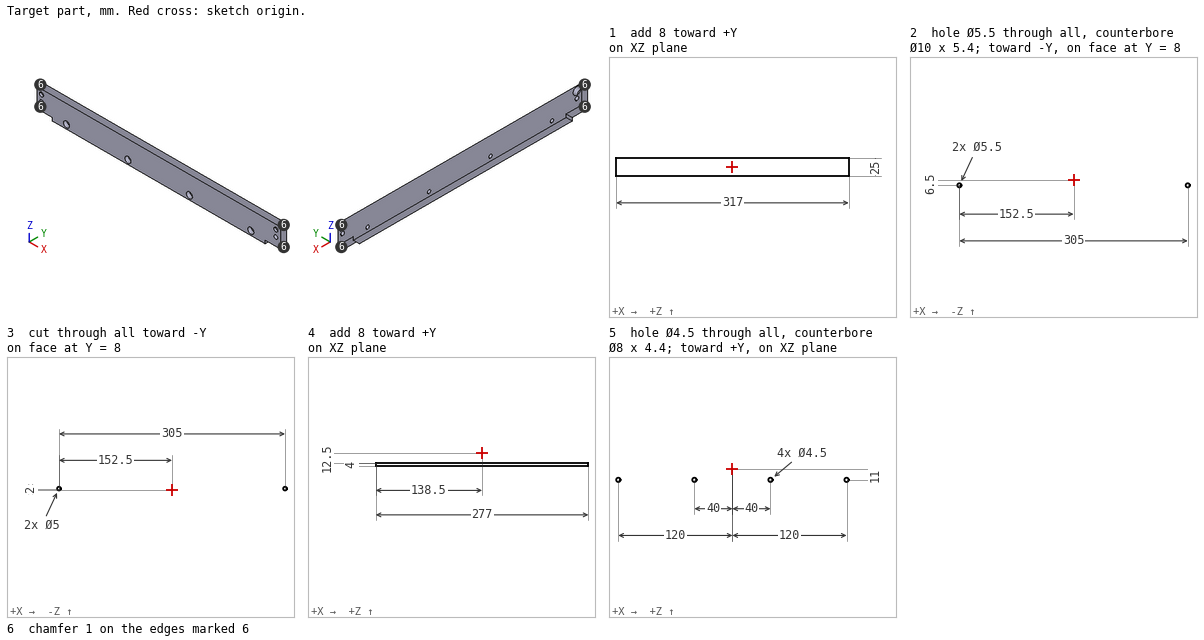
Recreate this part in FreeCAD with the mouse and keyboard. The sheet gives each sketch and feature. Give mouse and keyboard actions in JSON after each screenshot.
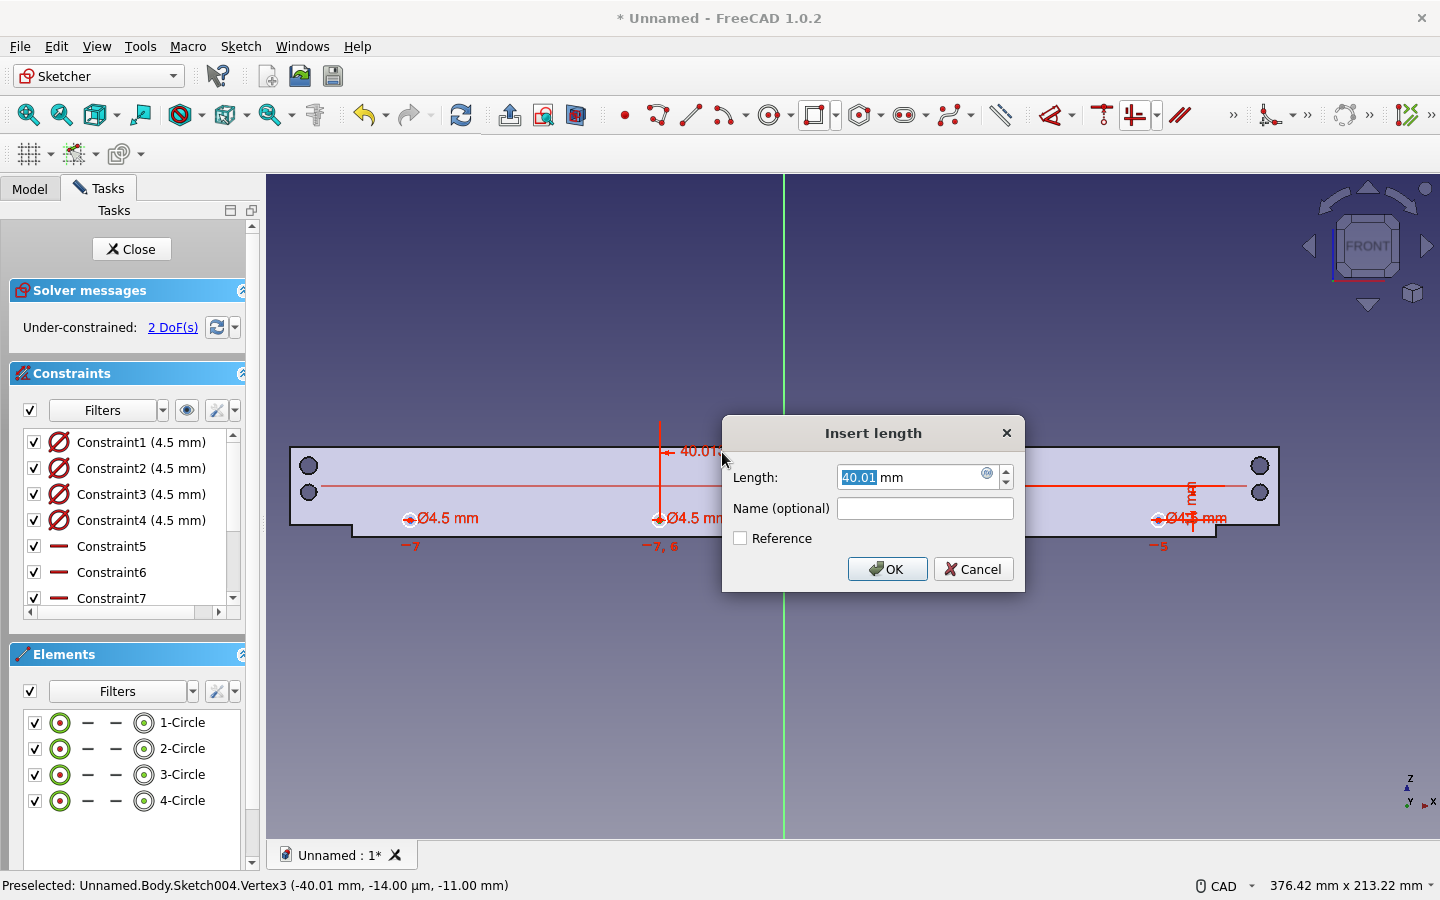
{"action": "type", "text": "40"}
{"action": "key", "text": "Return"}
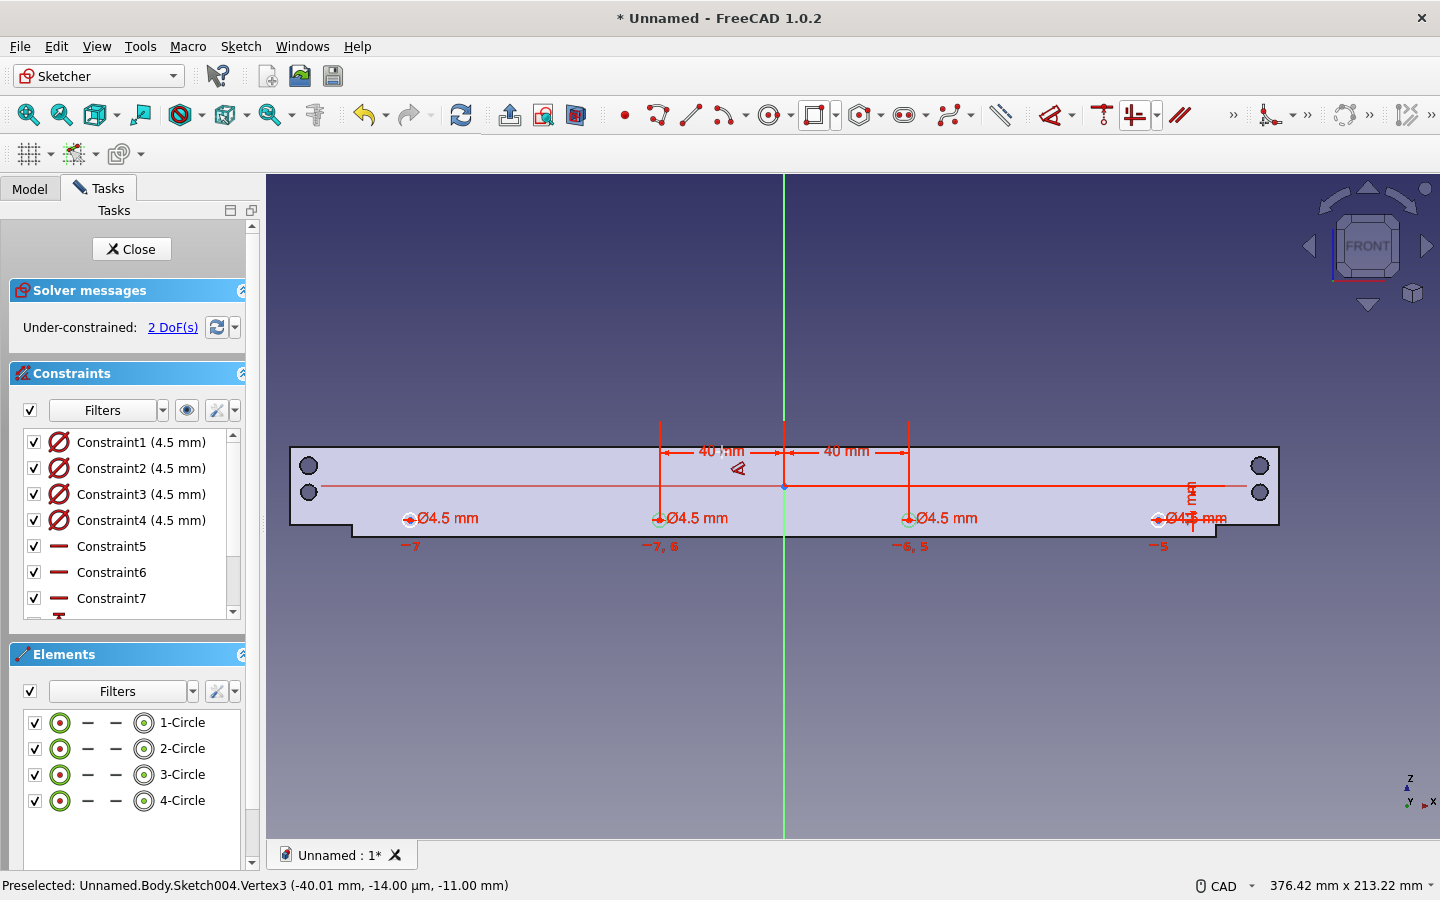
{"action": "left_click", "coordinate": [1159, 520]}
{"action": "left_click", "coordinate": [971, 452]}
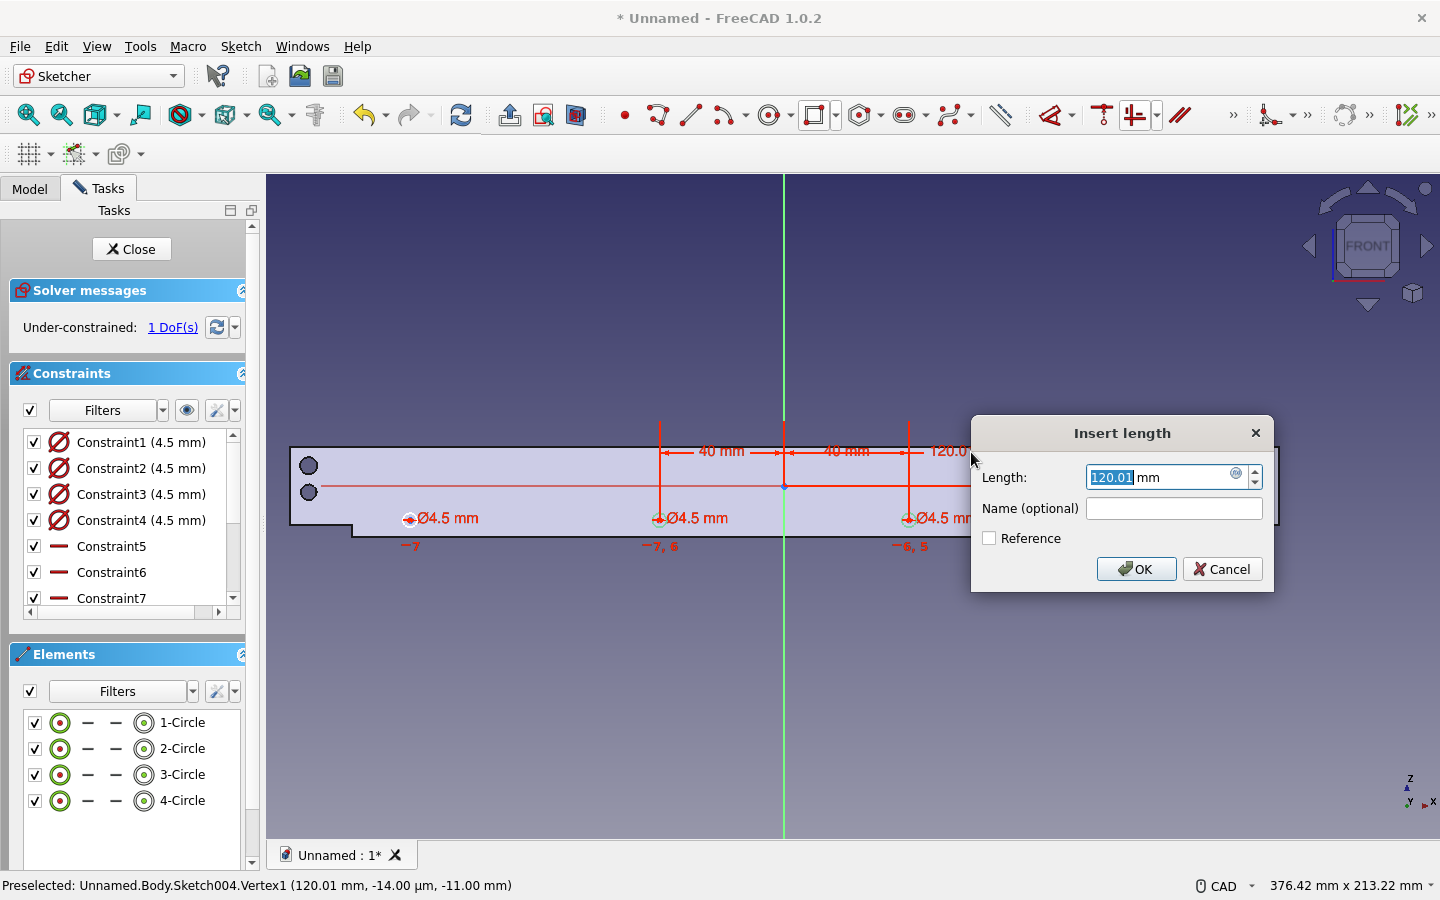
{"action": "type", "text": "120"}
{"action": "key", "text": "Return"}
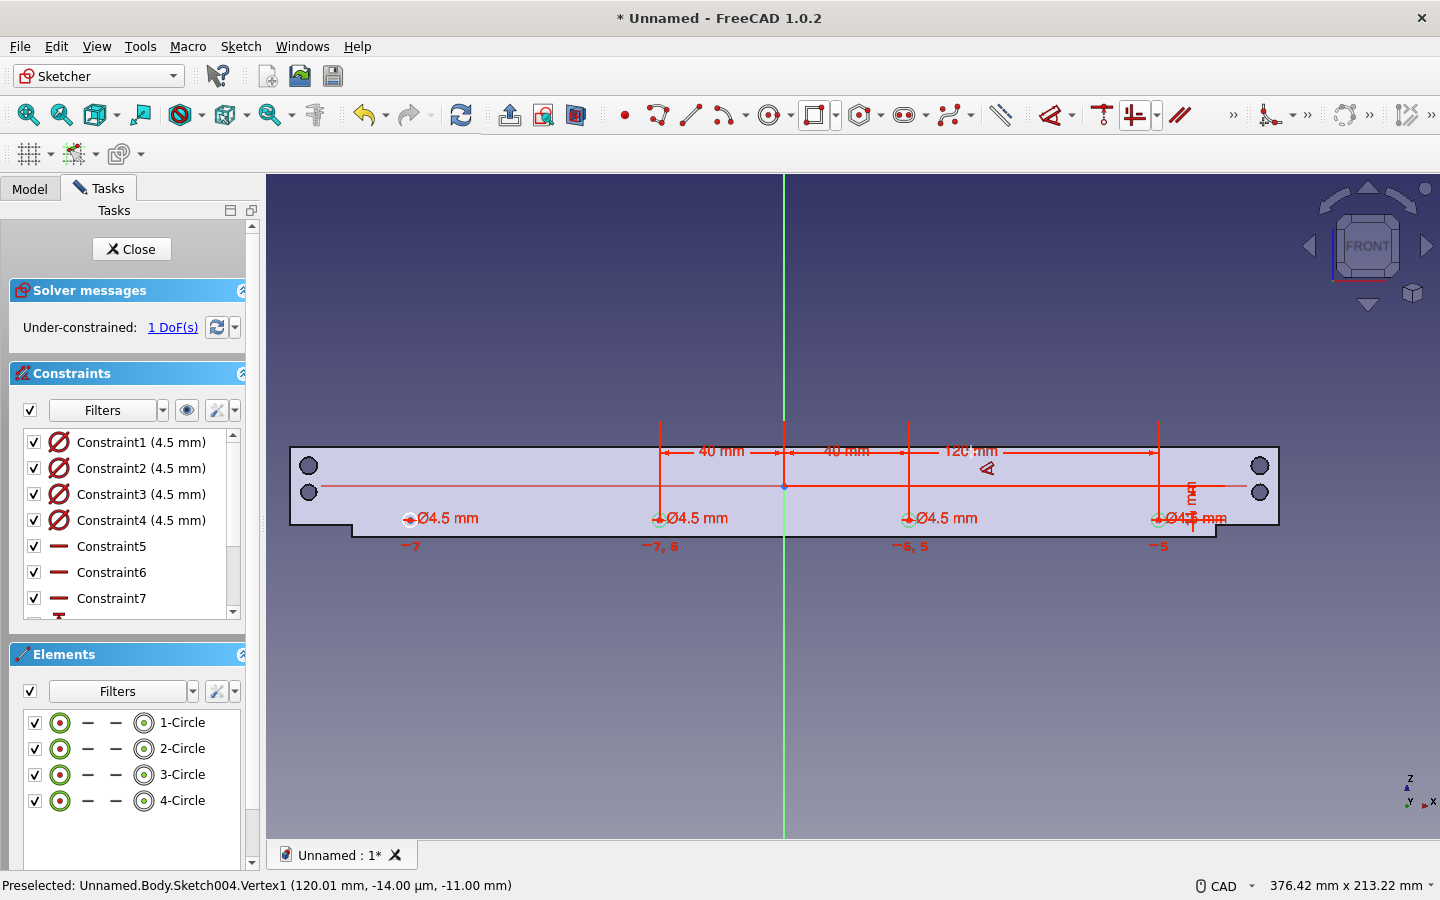
{"action": "left_click", "coordinate": [410, 520]}
{"action": "left_click", "coordinate": [597, 452]}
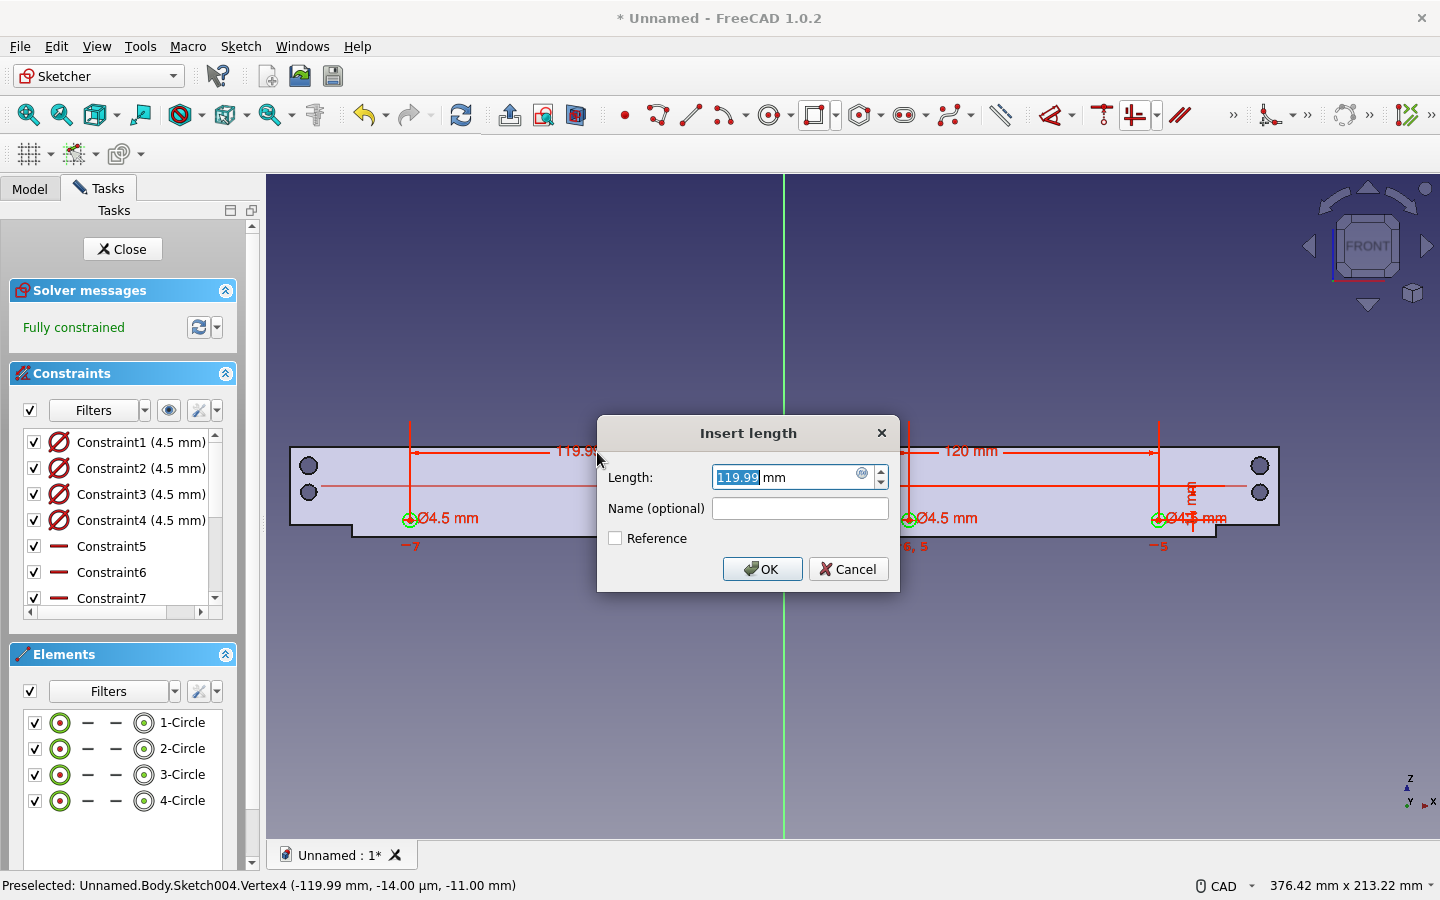
{"action": "type", "text": "120"}
{"action": "key", "text": "Return"}
{"action": "key", "text": "Escape"}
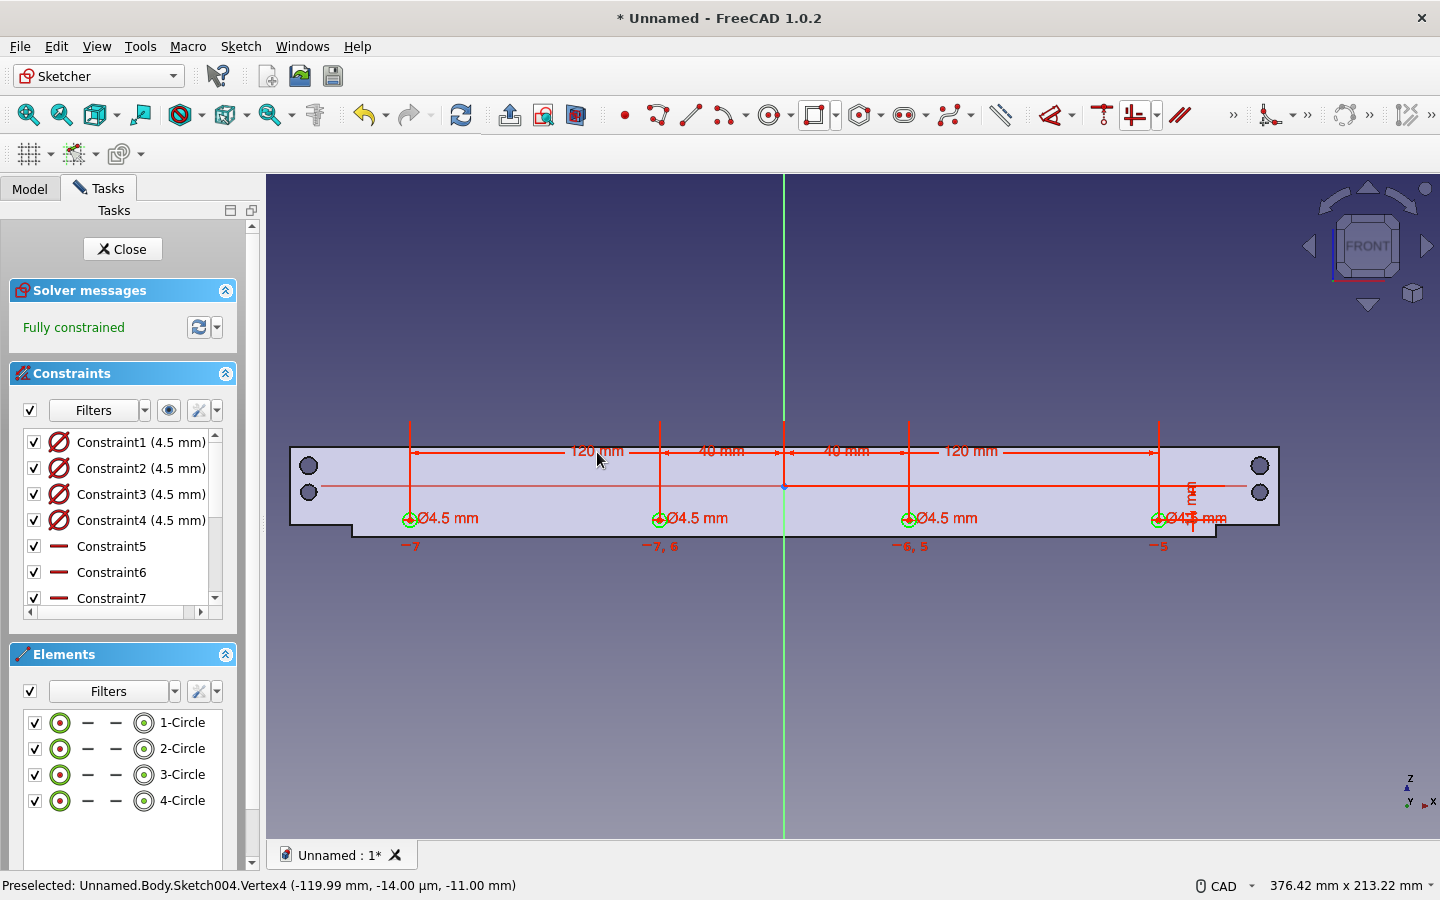
{"action": "left_click", "coordinate": [123, 249]}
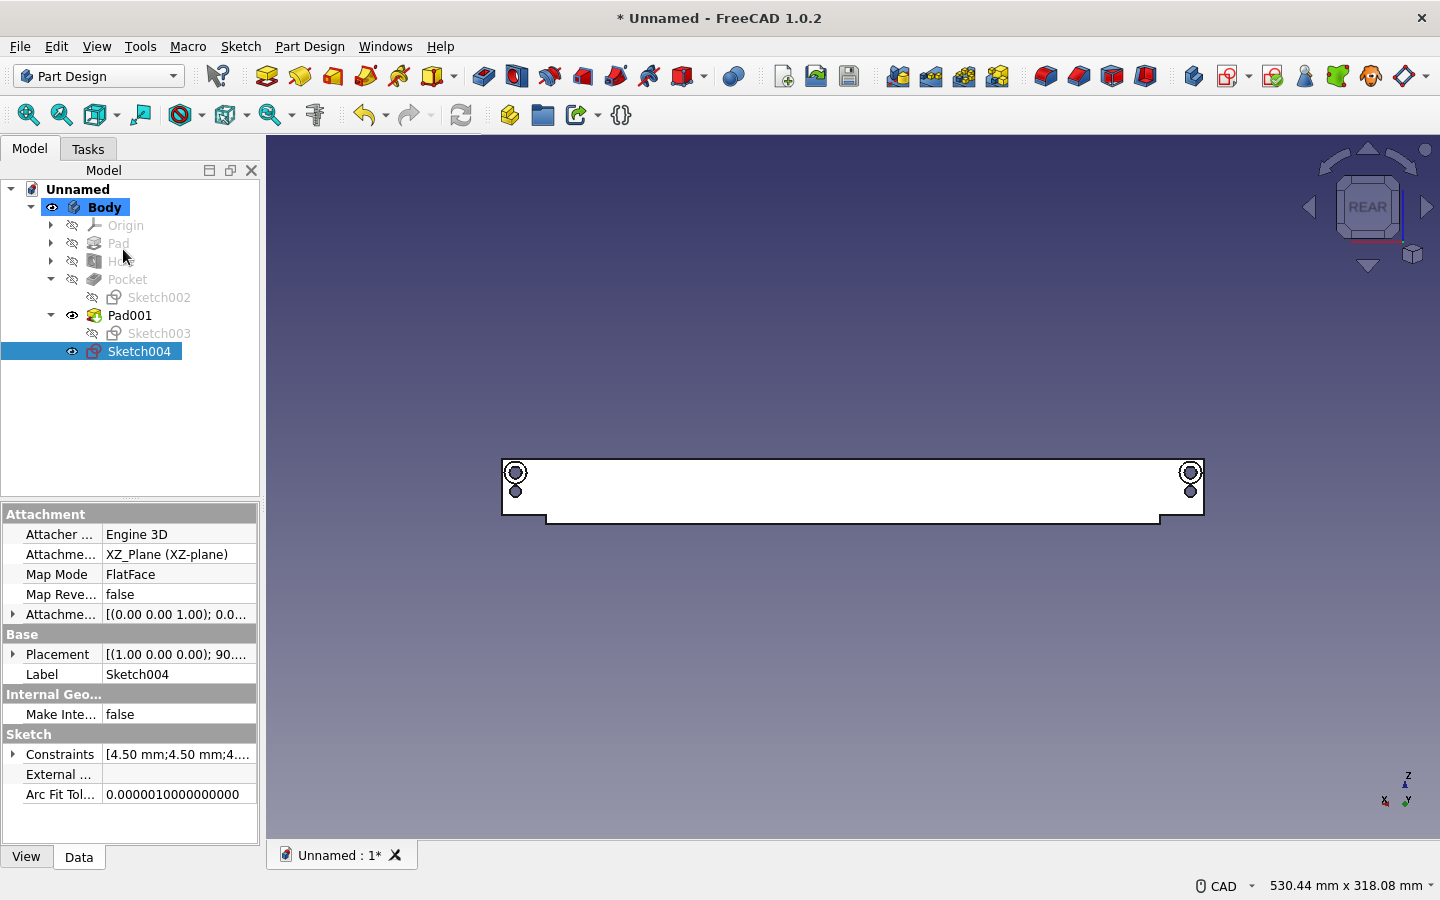
{"action": "left_click", "coordinate": [517, 76]}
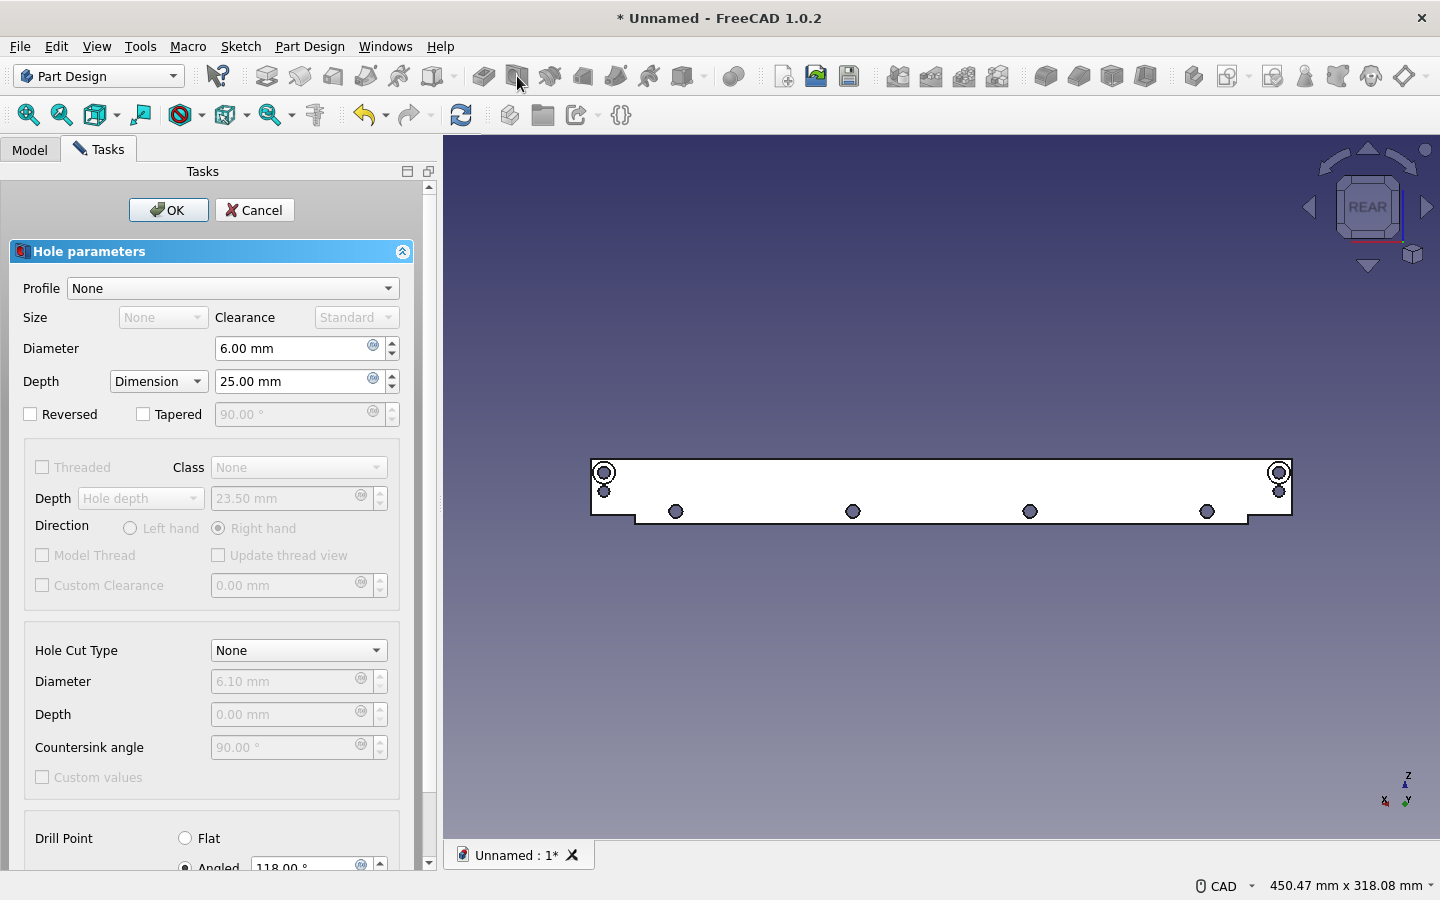
{"action": "triple_click", "coordinate": [300, 348]}